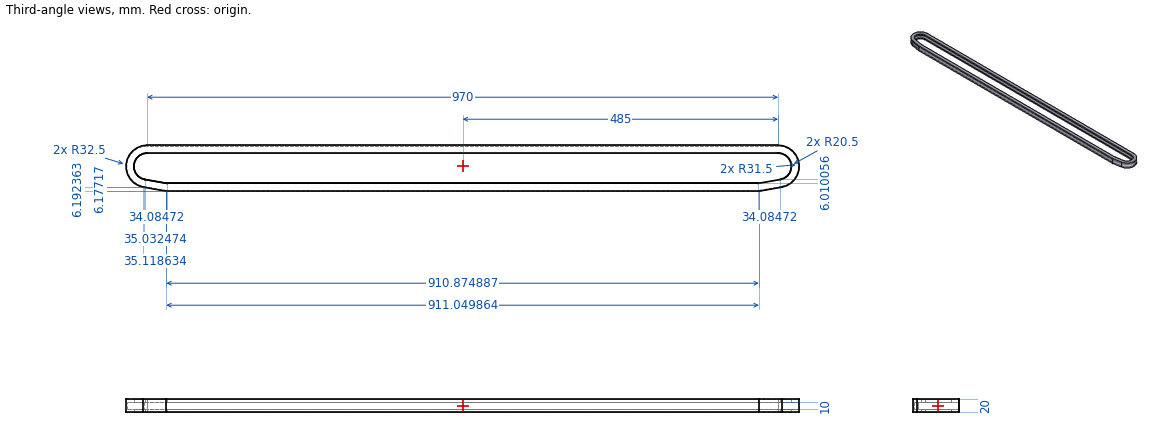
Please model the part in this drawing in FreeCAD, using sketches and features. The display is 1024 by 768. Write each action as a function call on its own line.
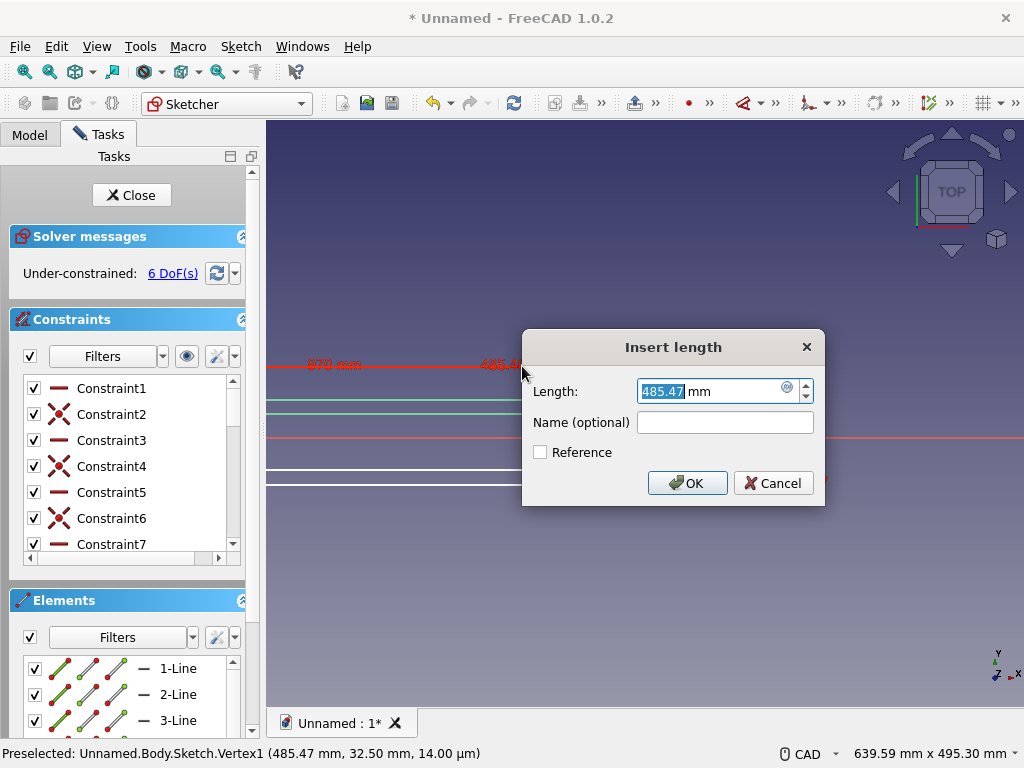
text(485)
key(Return)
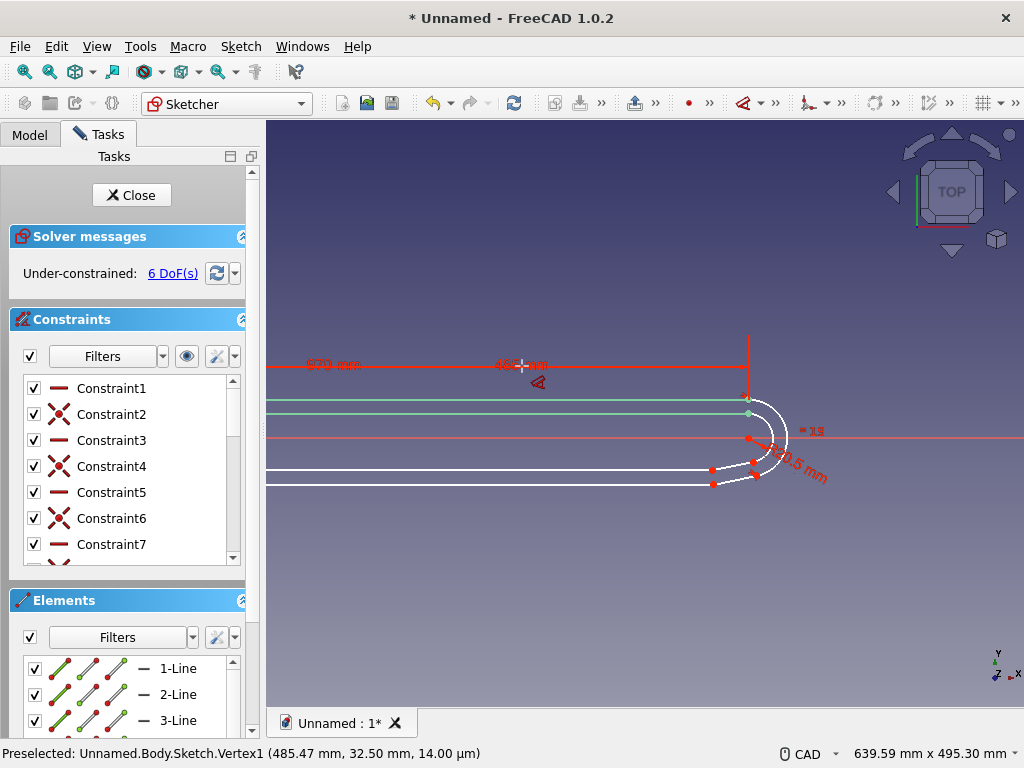
scroll(750, 401, down, 6)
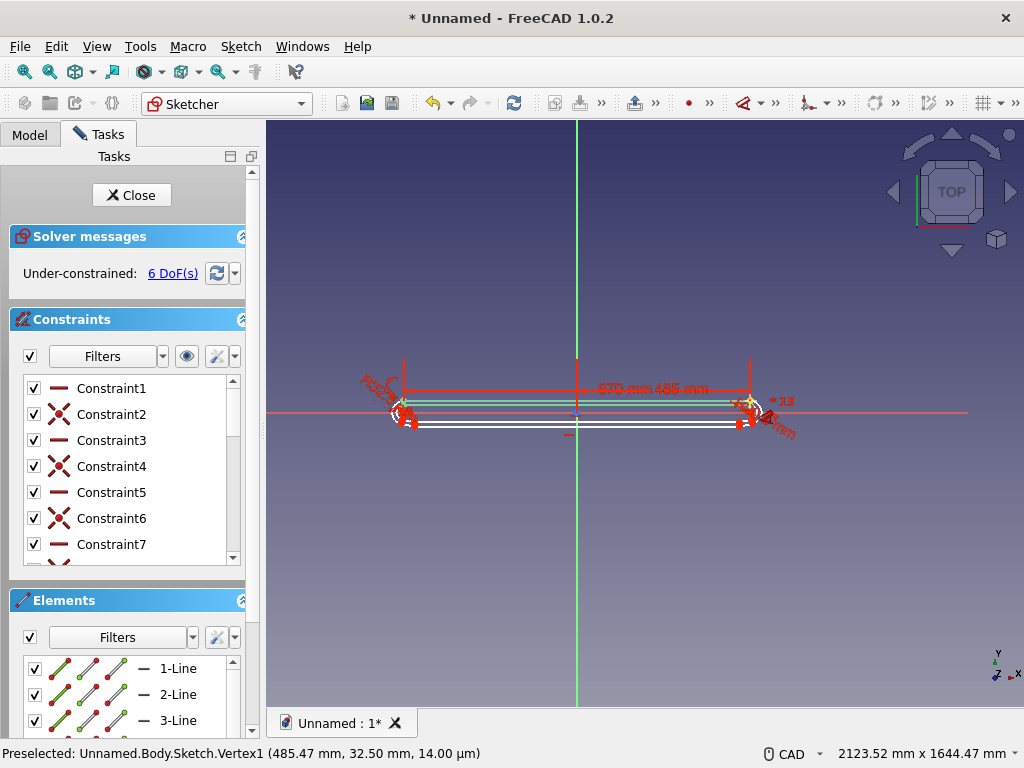
scroll(405, 425, up, 15)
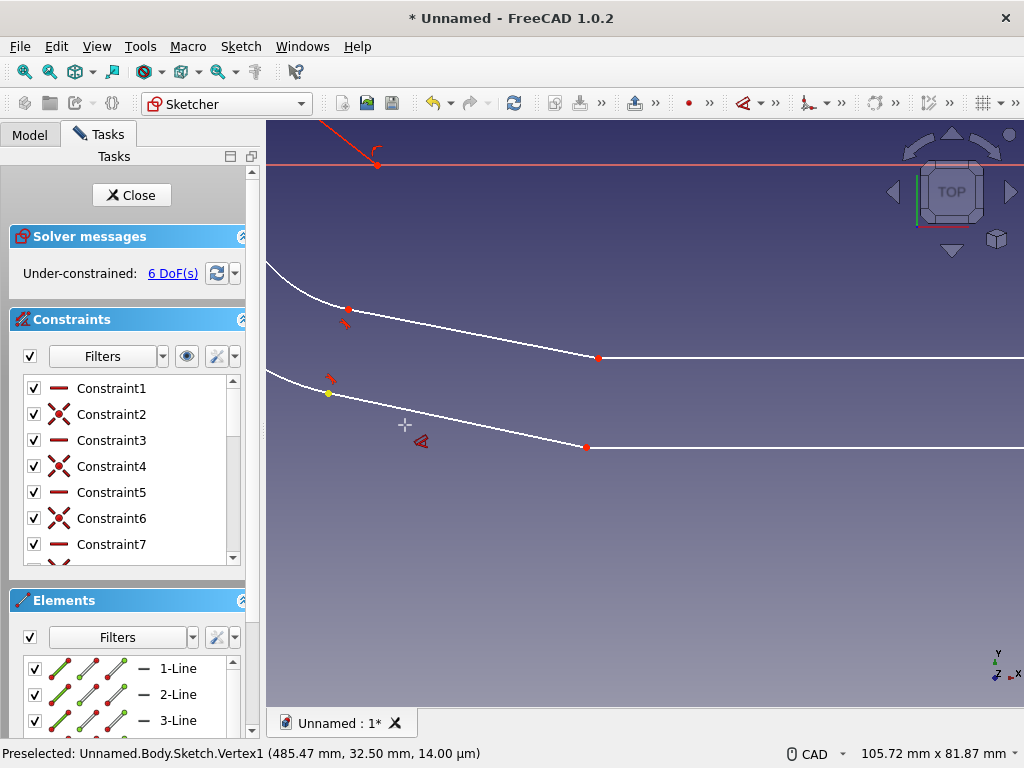
click(406, 410)
click(295, 420)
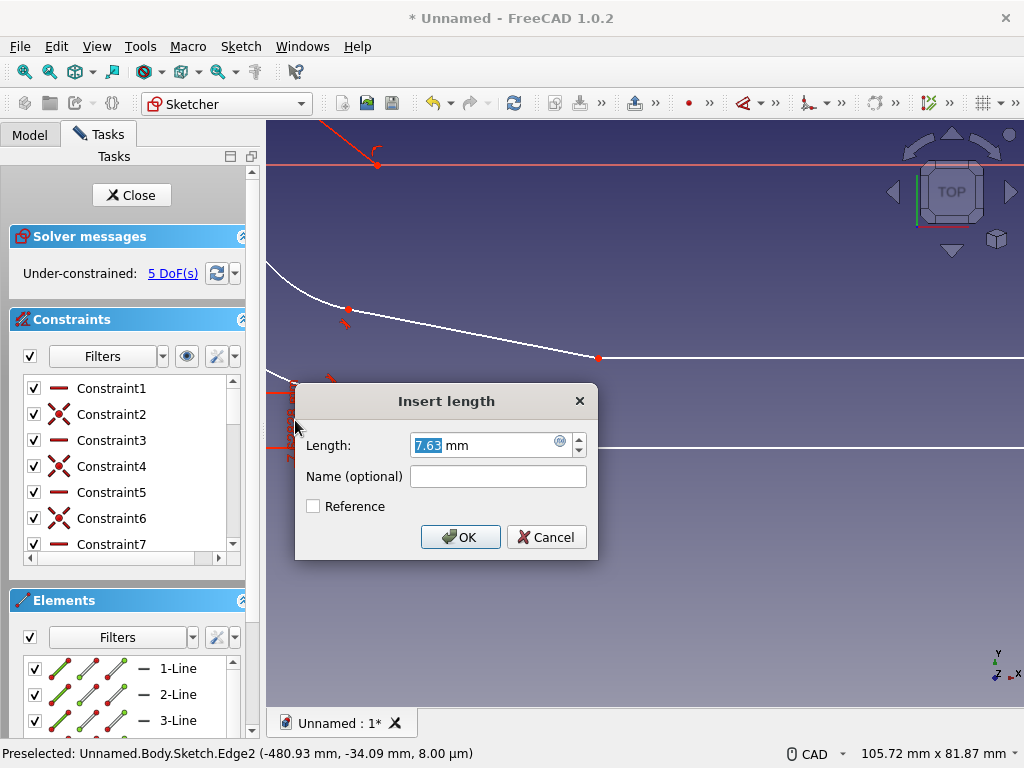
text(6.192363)
key(Return)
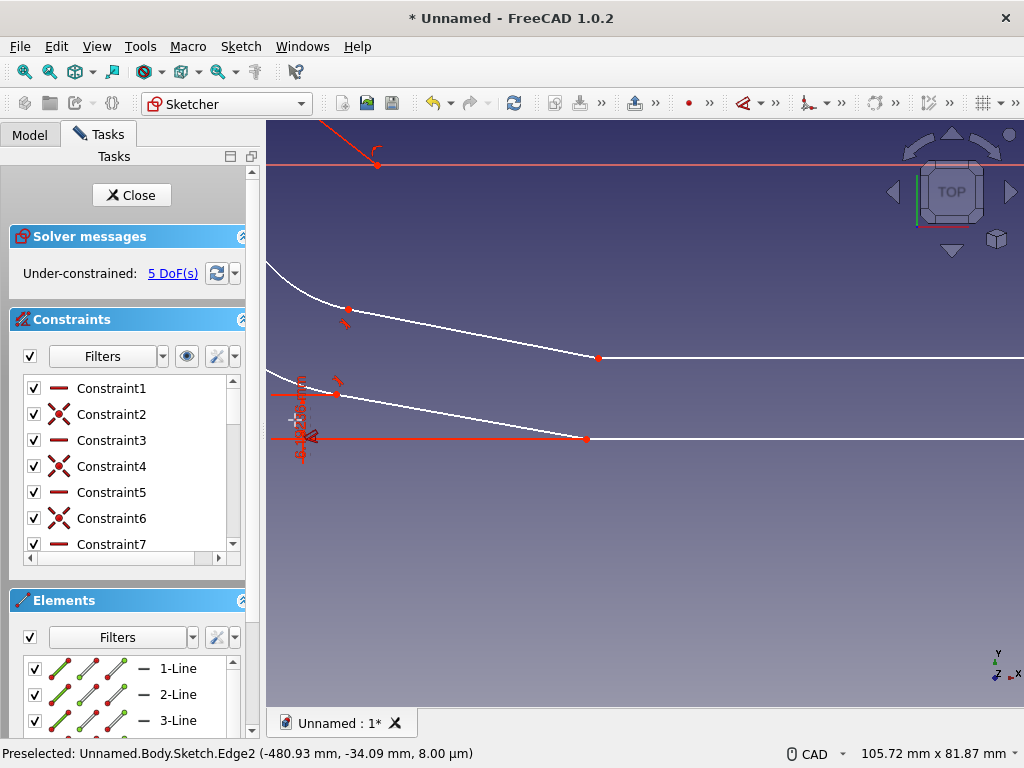
scroll(405, 425, down, 15)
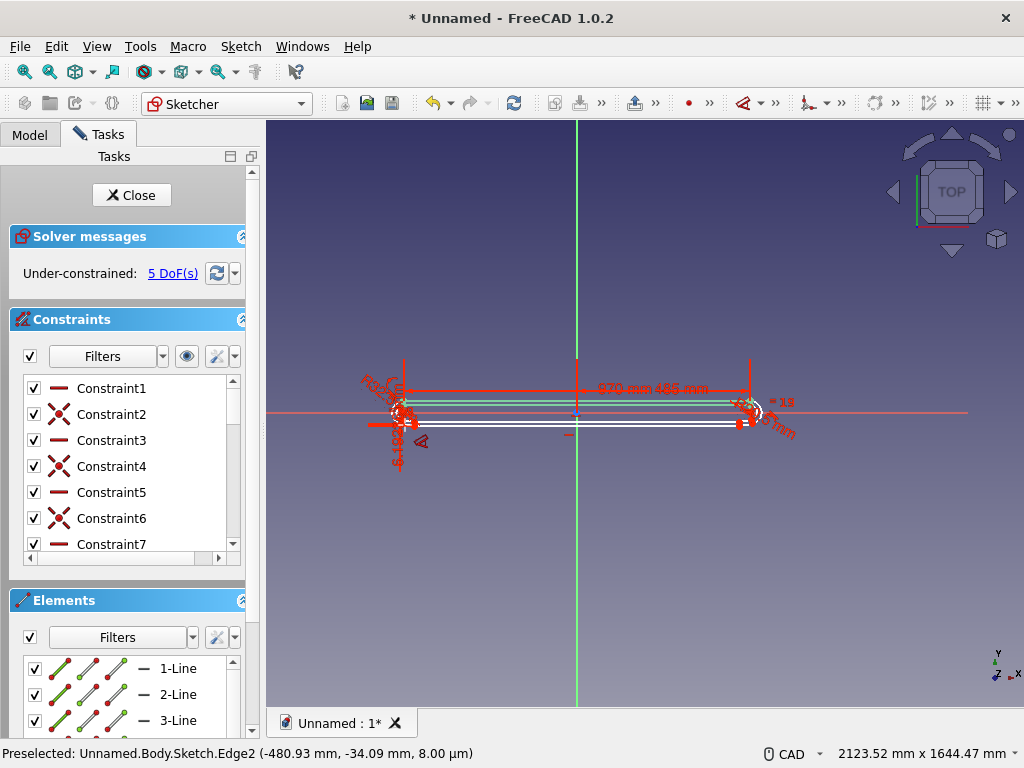
scroll(748, 420, up, 7)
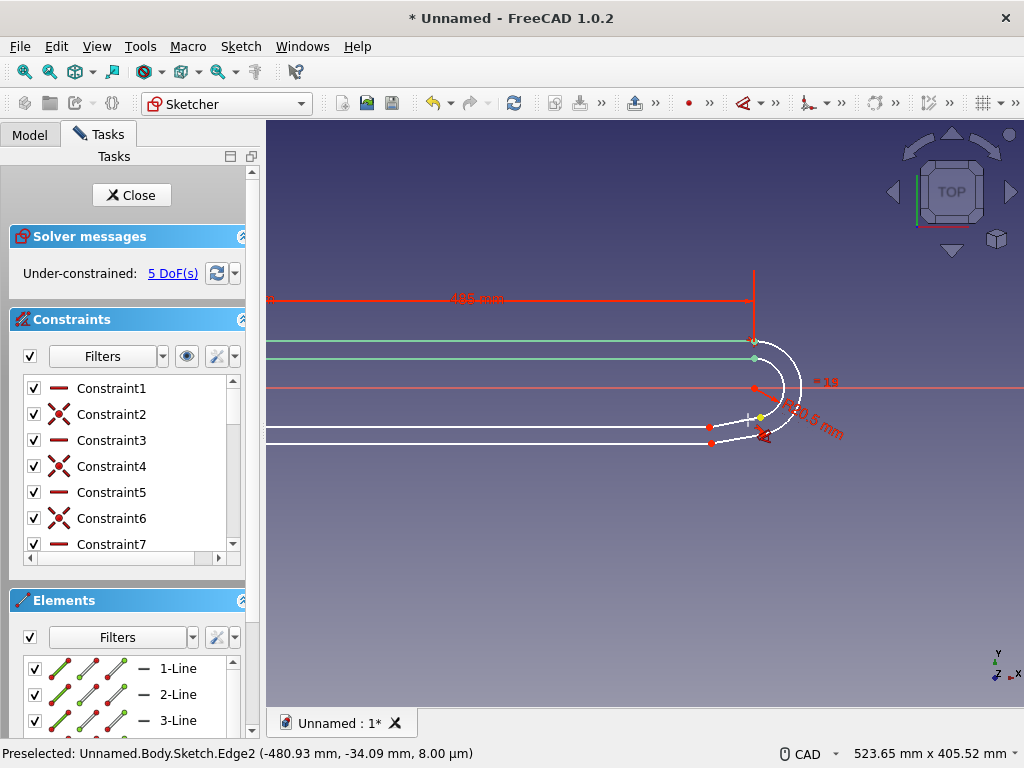
click(745, 420)
click(735, 461)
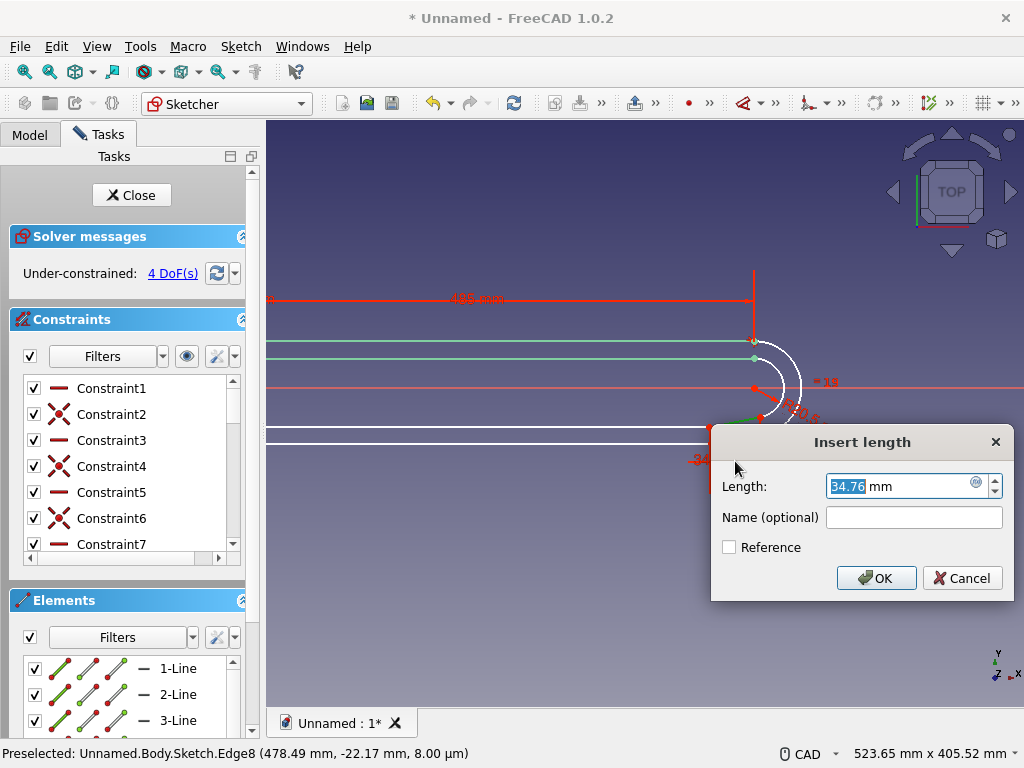
text(34.08472)
key(Return)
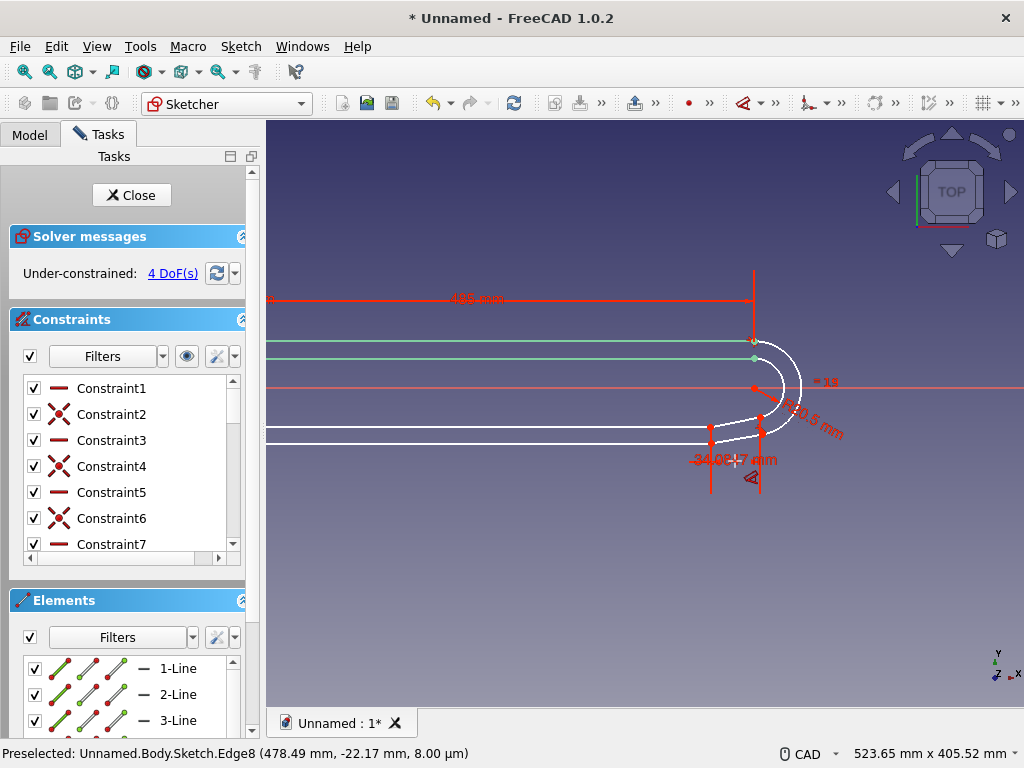
scroll(745, 420, up, 8)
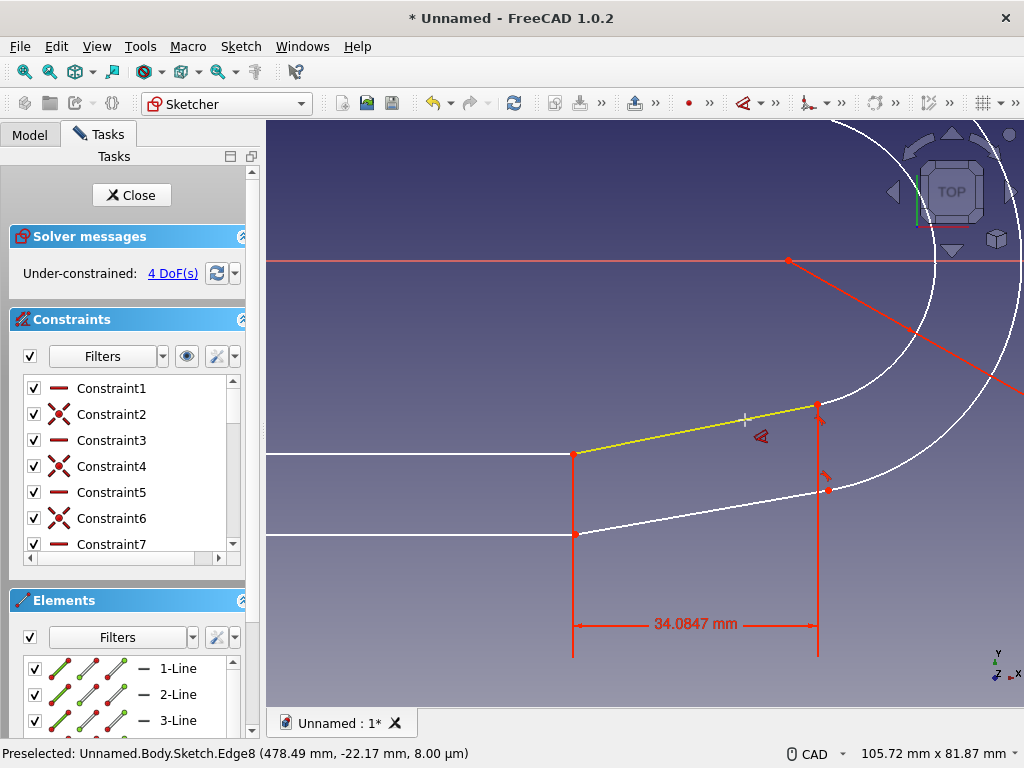
click(744, 420)
click(852, 429)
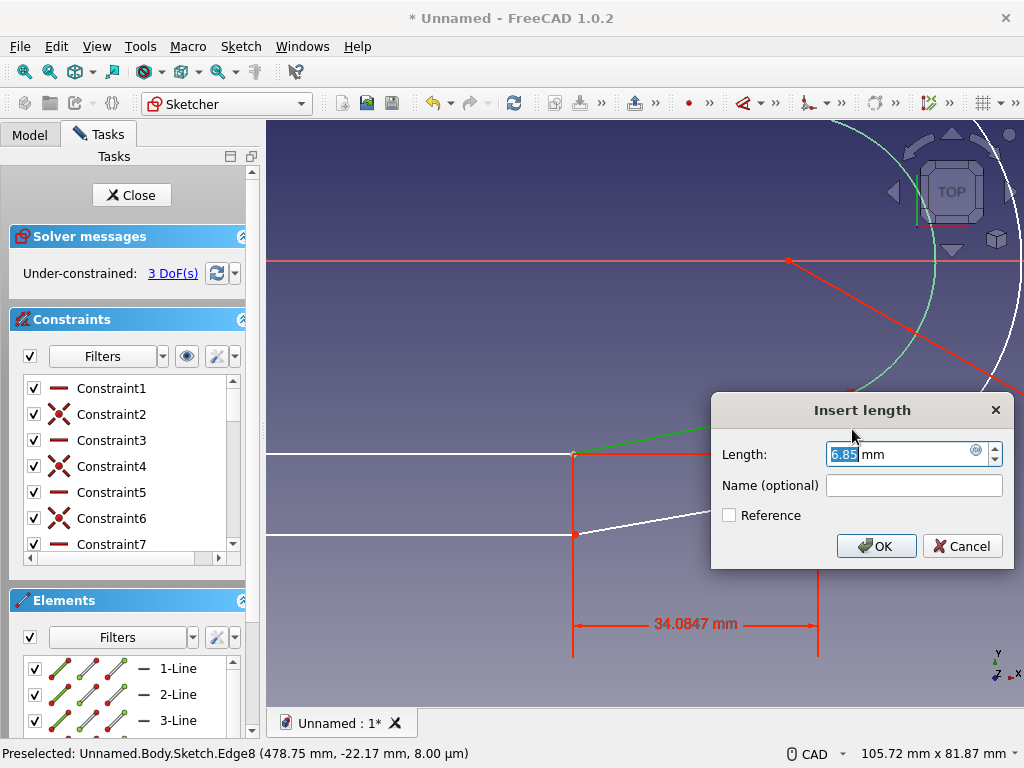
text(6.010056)
key(Return)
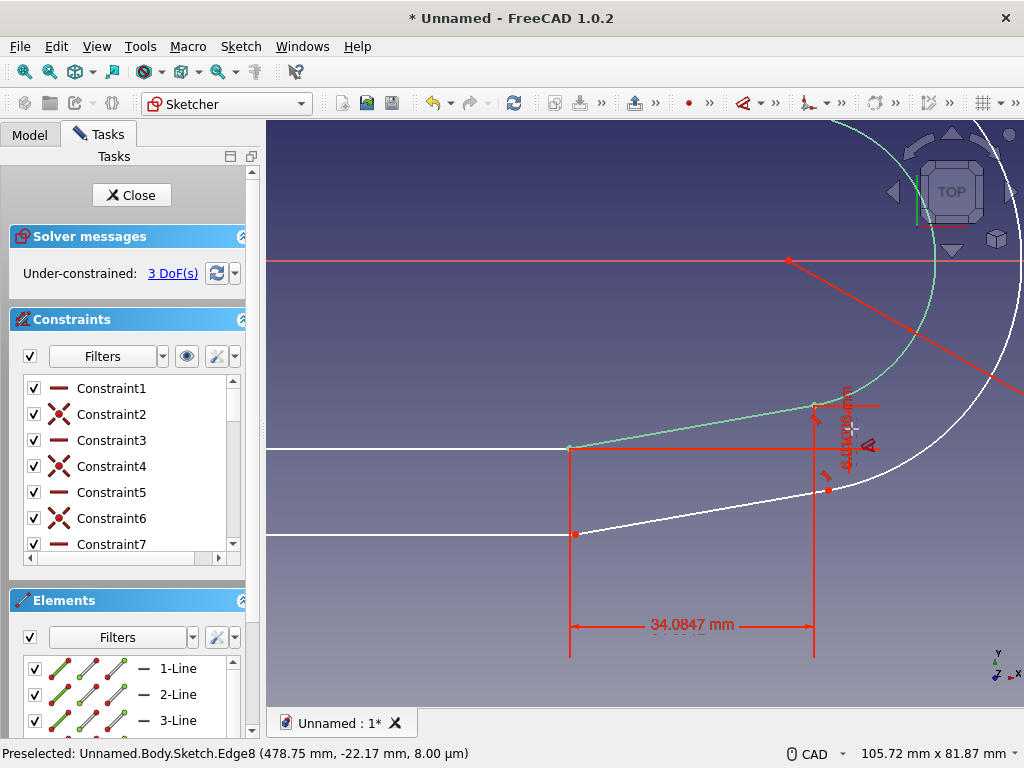
scroll(748, 420, down, 15)